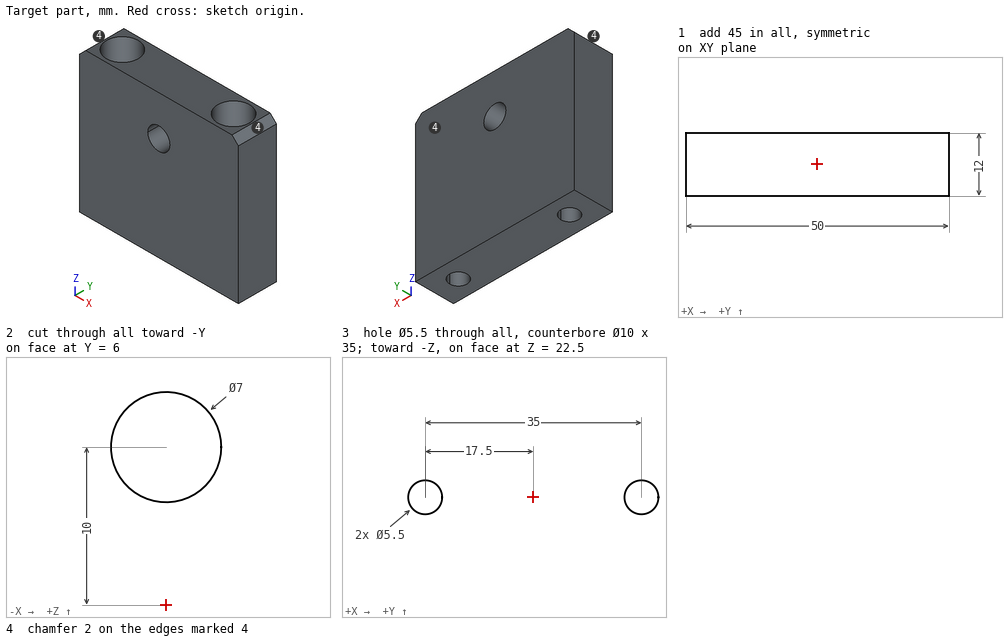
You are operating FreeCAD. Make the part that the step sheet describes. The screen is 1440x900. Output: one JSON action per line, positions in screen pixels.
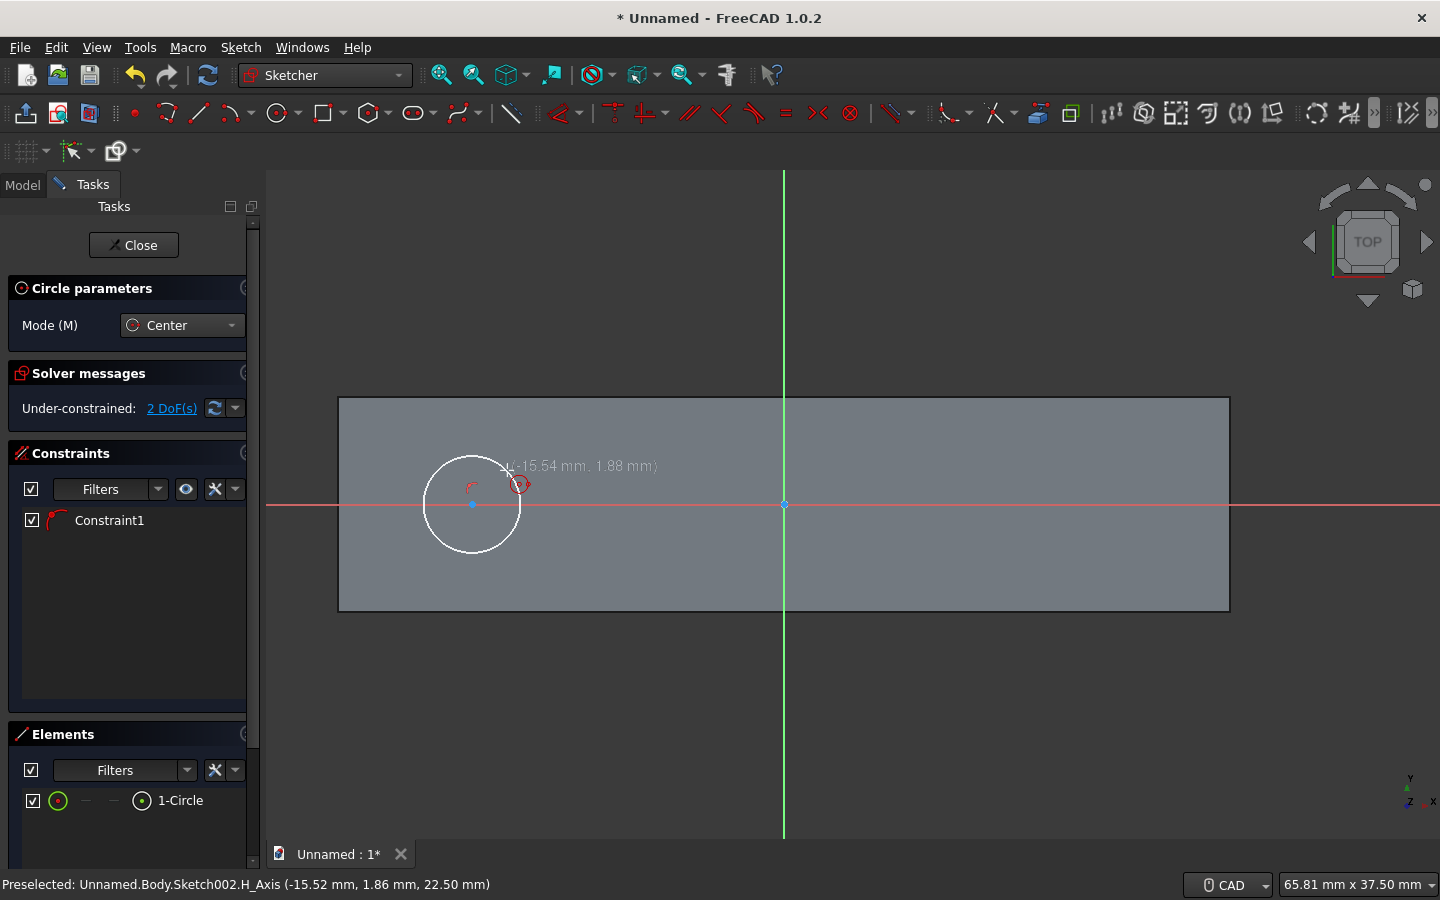
{"action": "left_click", "coordinate": [1096, 504]}
{"action": "left_click", "coordinate": [1131, 470]}
{"action": "key", "text": "Escape"}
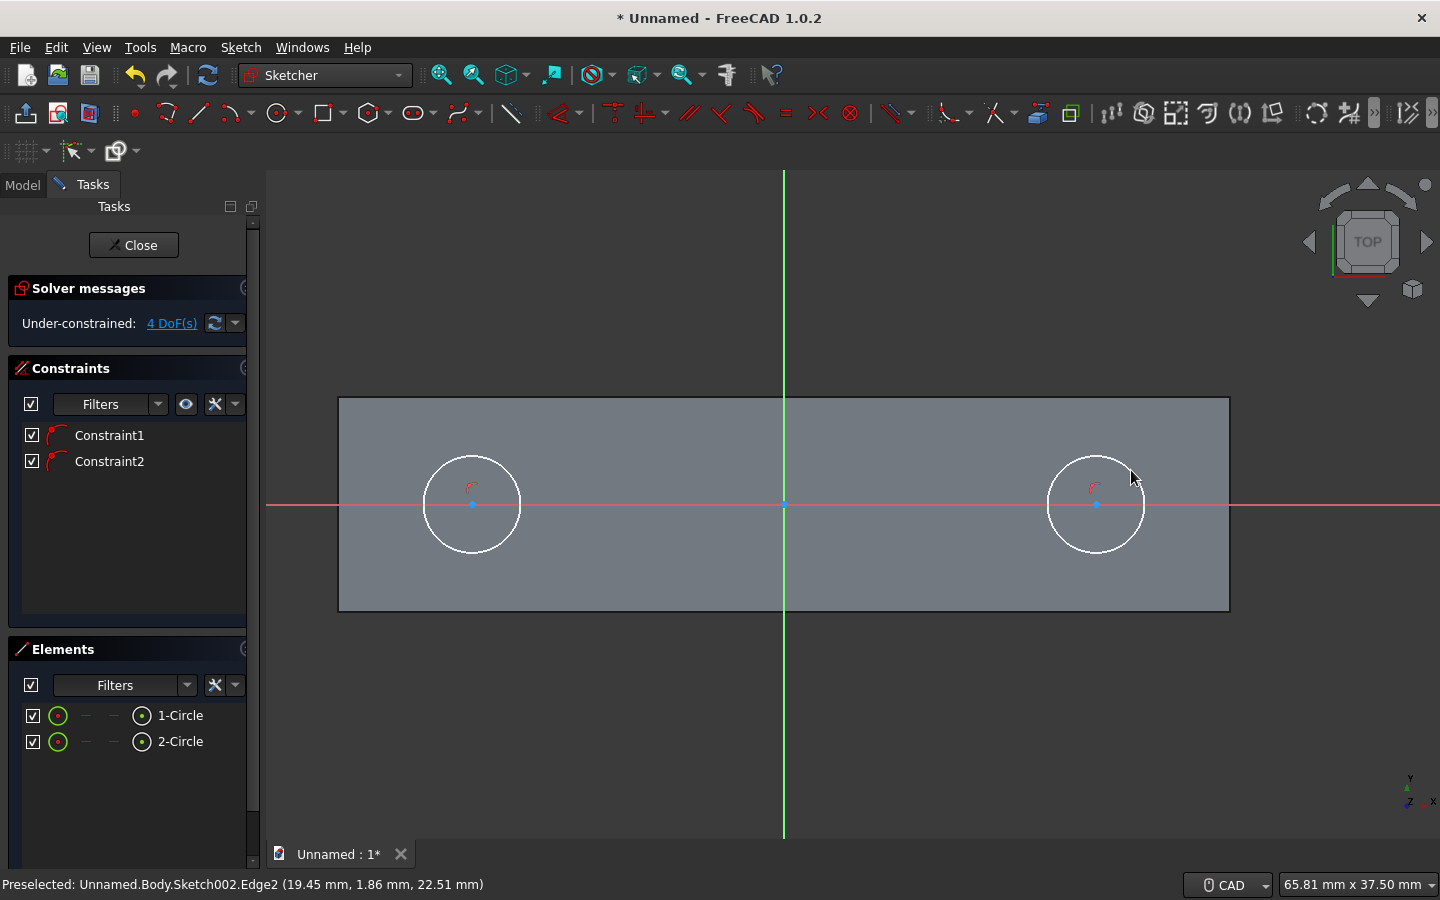
{"action": "left_click", "coordinate": [506, 470]}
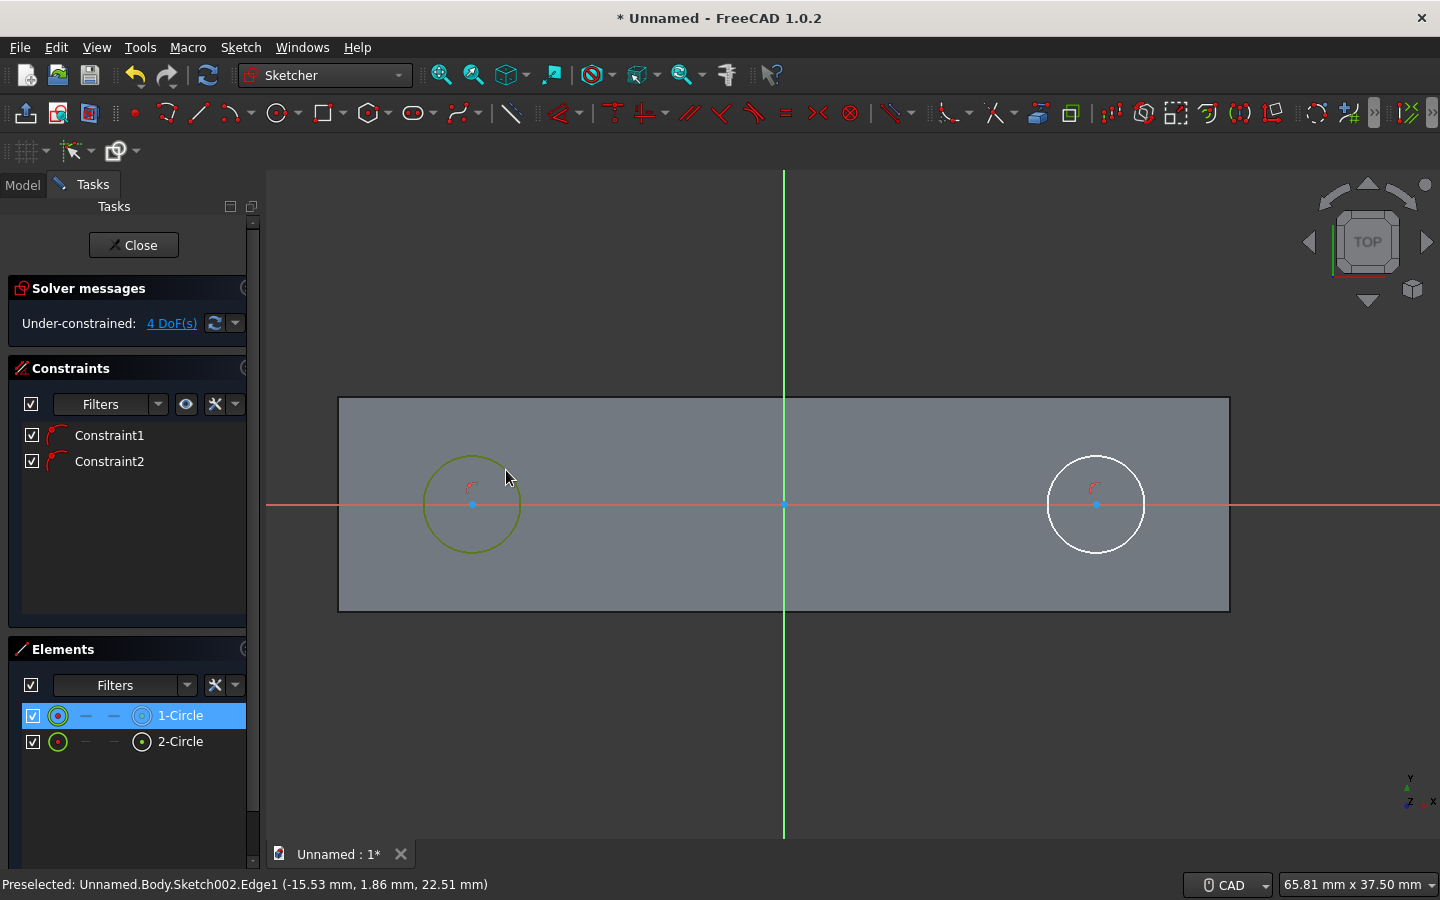
{"action": "left_click", "coordinate": [1130, 470]}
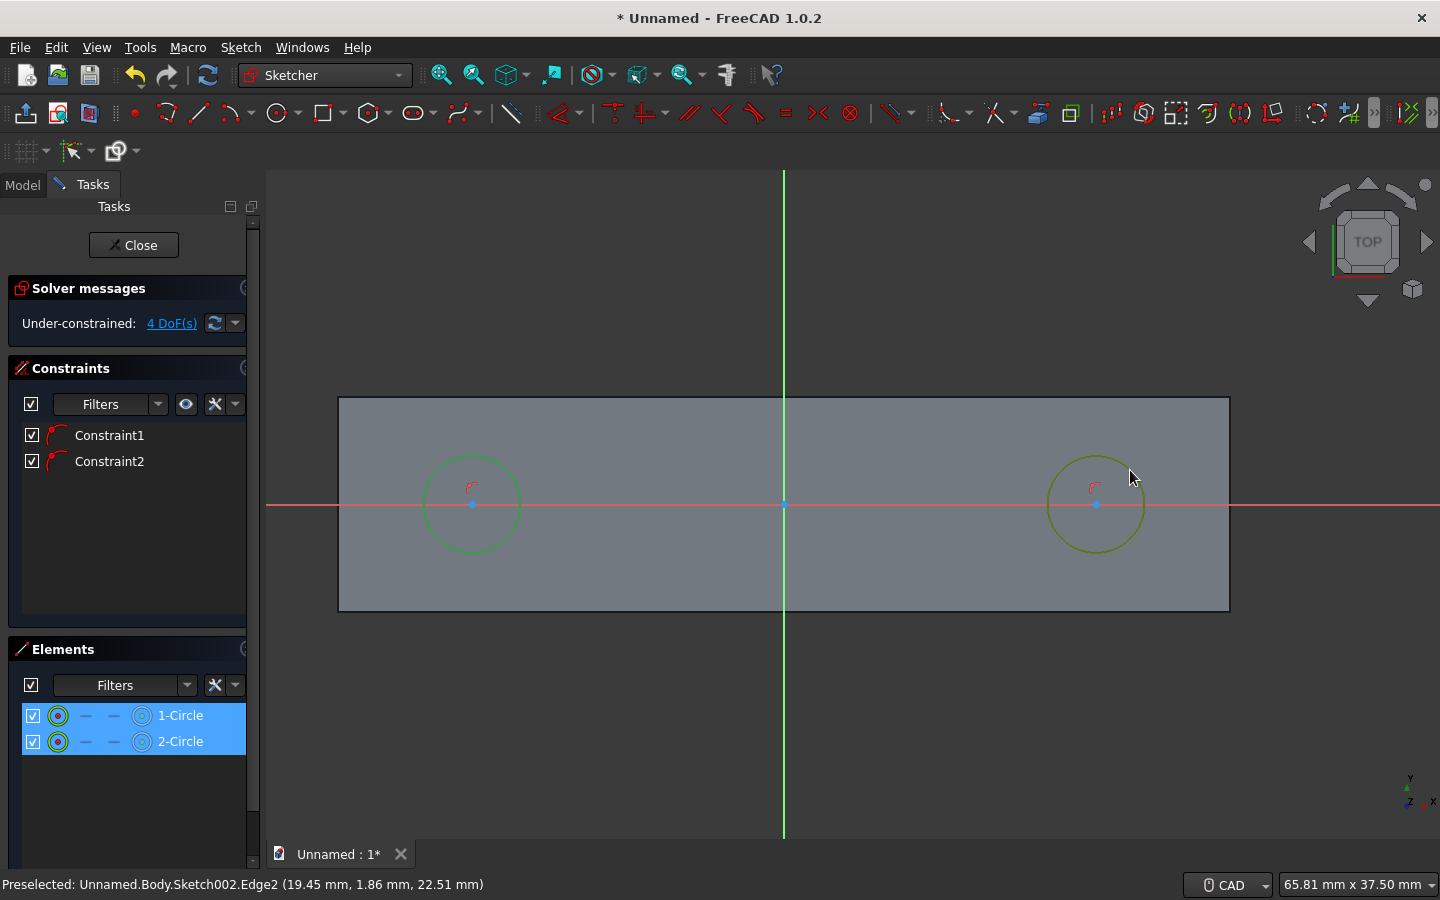
{"action": "key", "text": "e"}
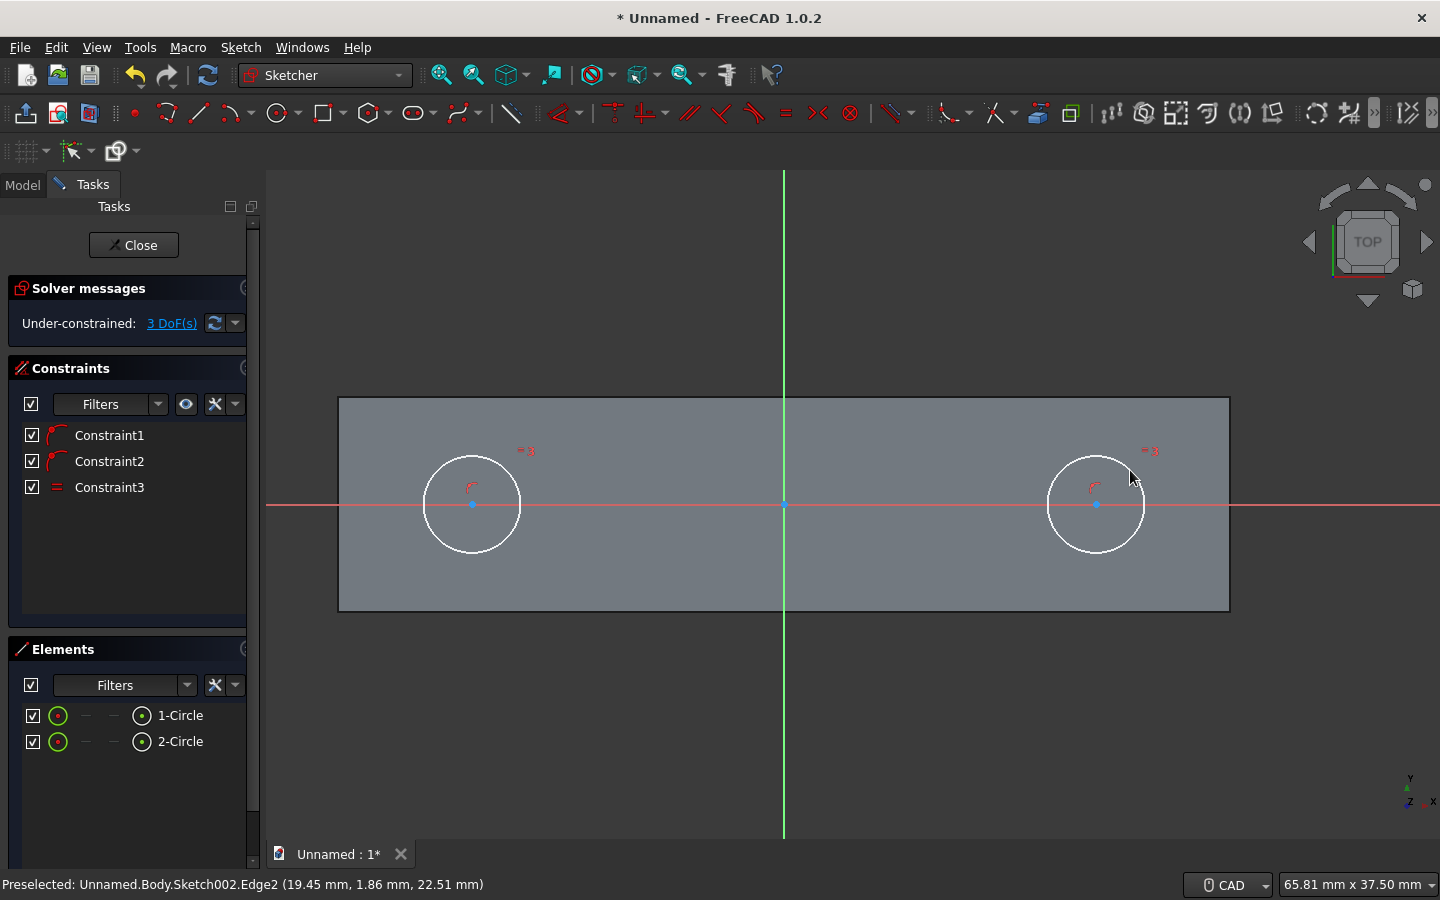
{"action": "left_click", "coordinate": [558, 114]}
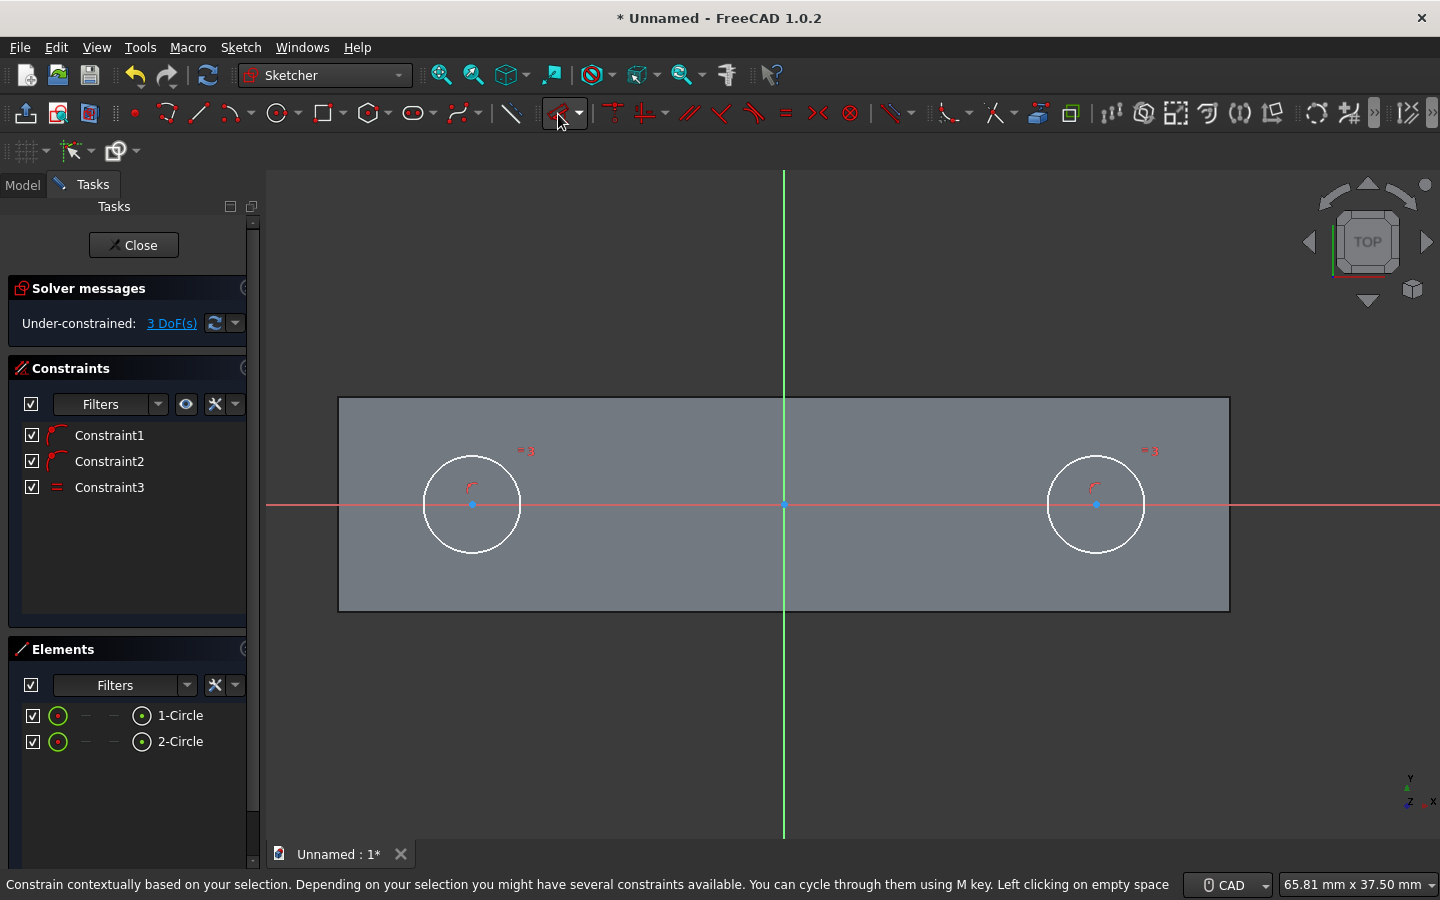
{"action": "left_click", "coordinate": [506, 470]}
{"action": "left_click", "coordinate": [528, 447]}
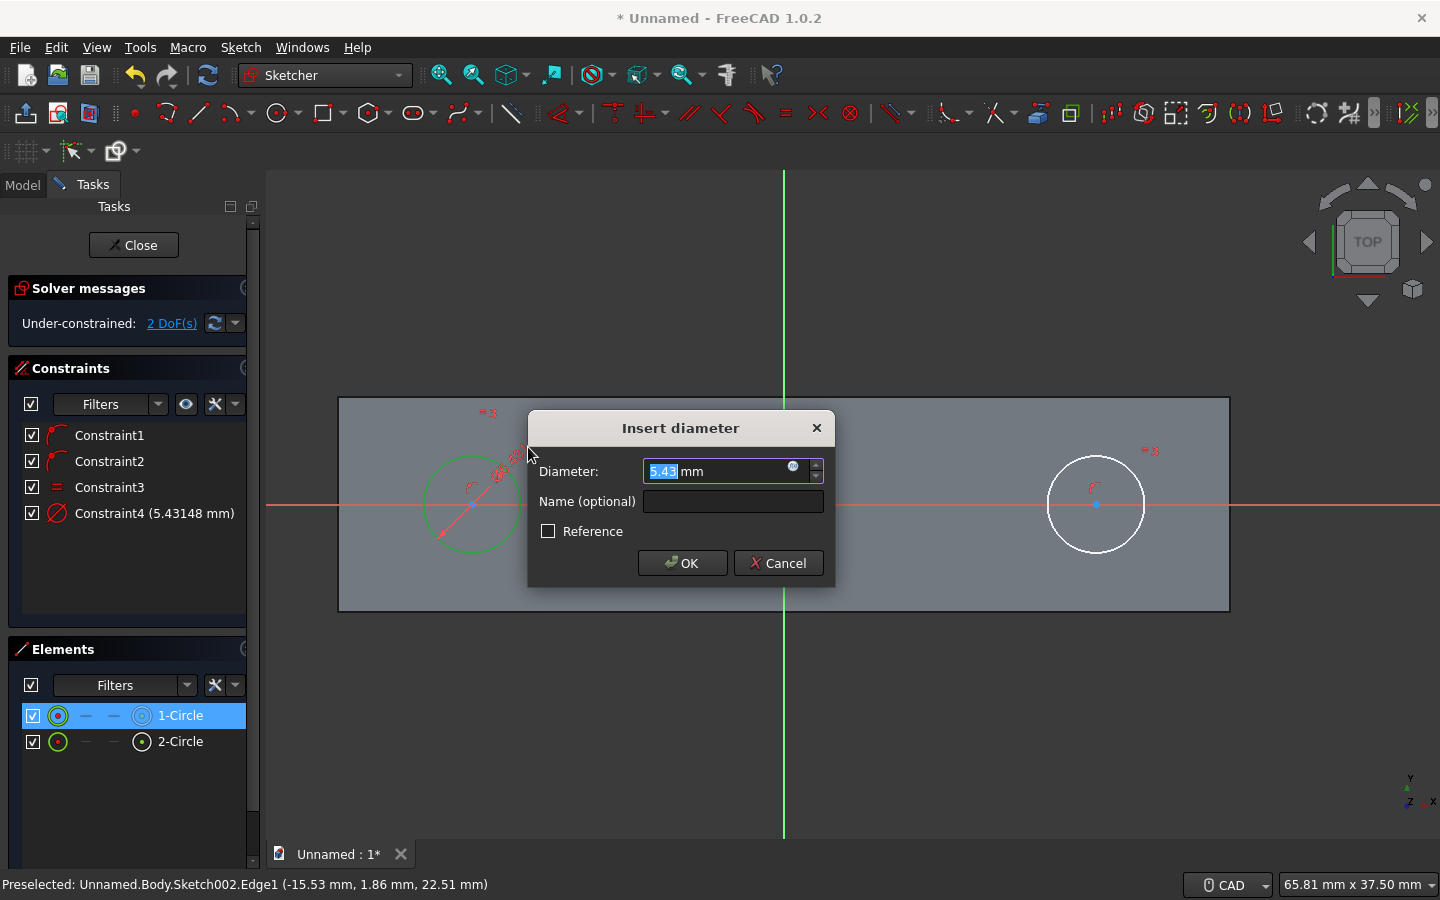
{"action": "type", "text": "5.5"}
{"action": "key", "text": "Return"}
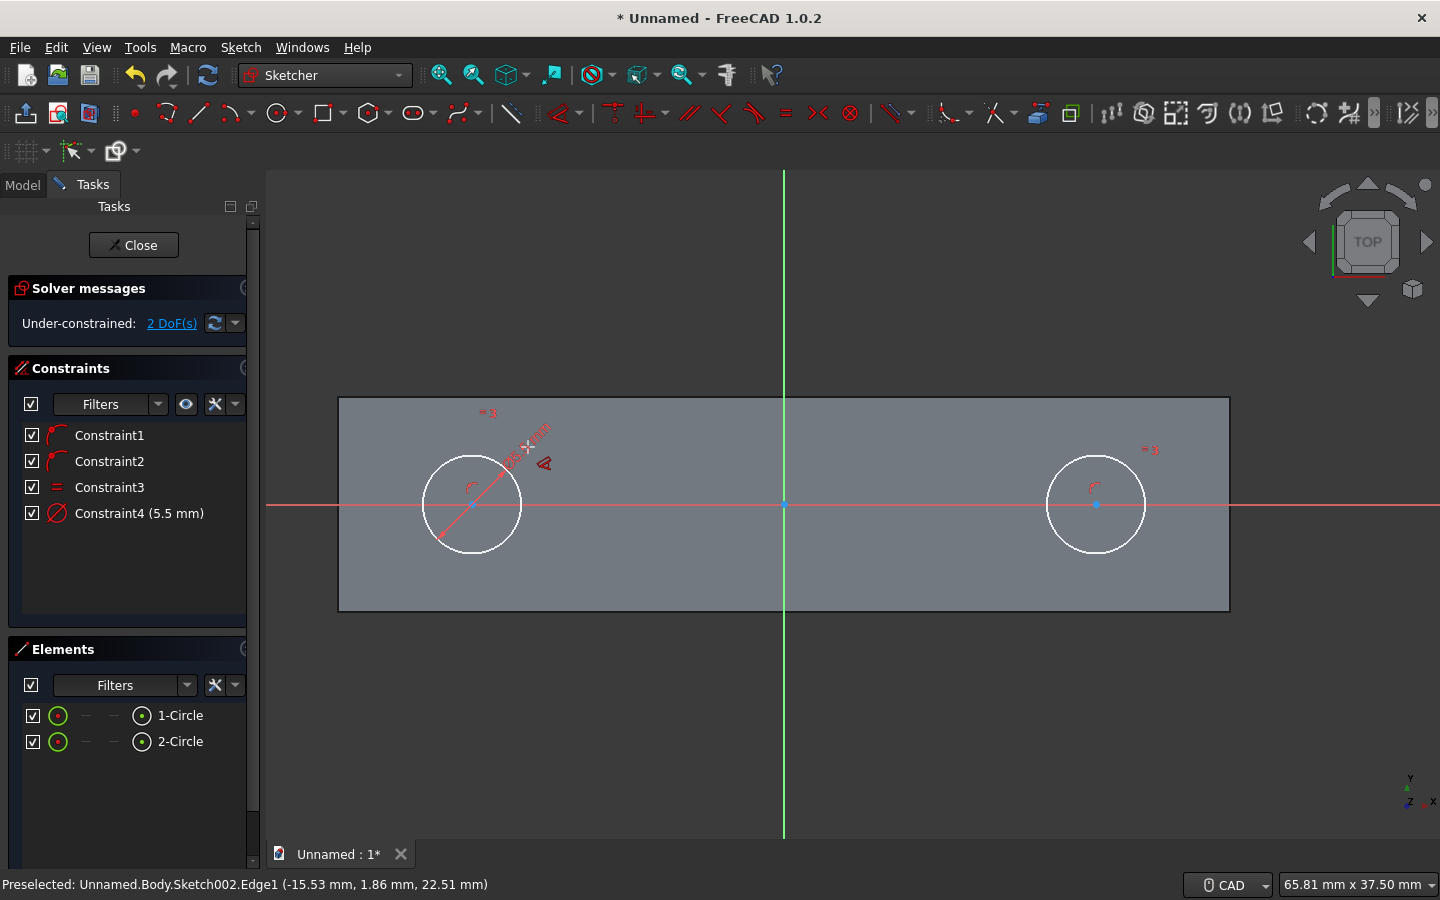
{"action": "left_click", "coordinate": [472, 504]}